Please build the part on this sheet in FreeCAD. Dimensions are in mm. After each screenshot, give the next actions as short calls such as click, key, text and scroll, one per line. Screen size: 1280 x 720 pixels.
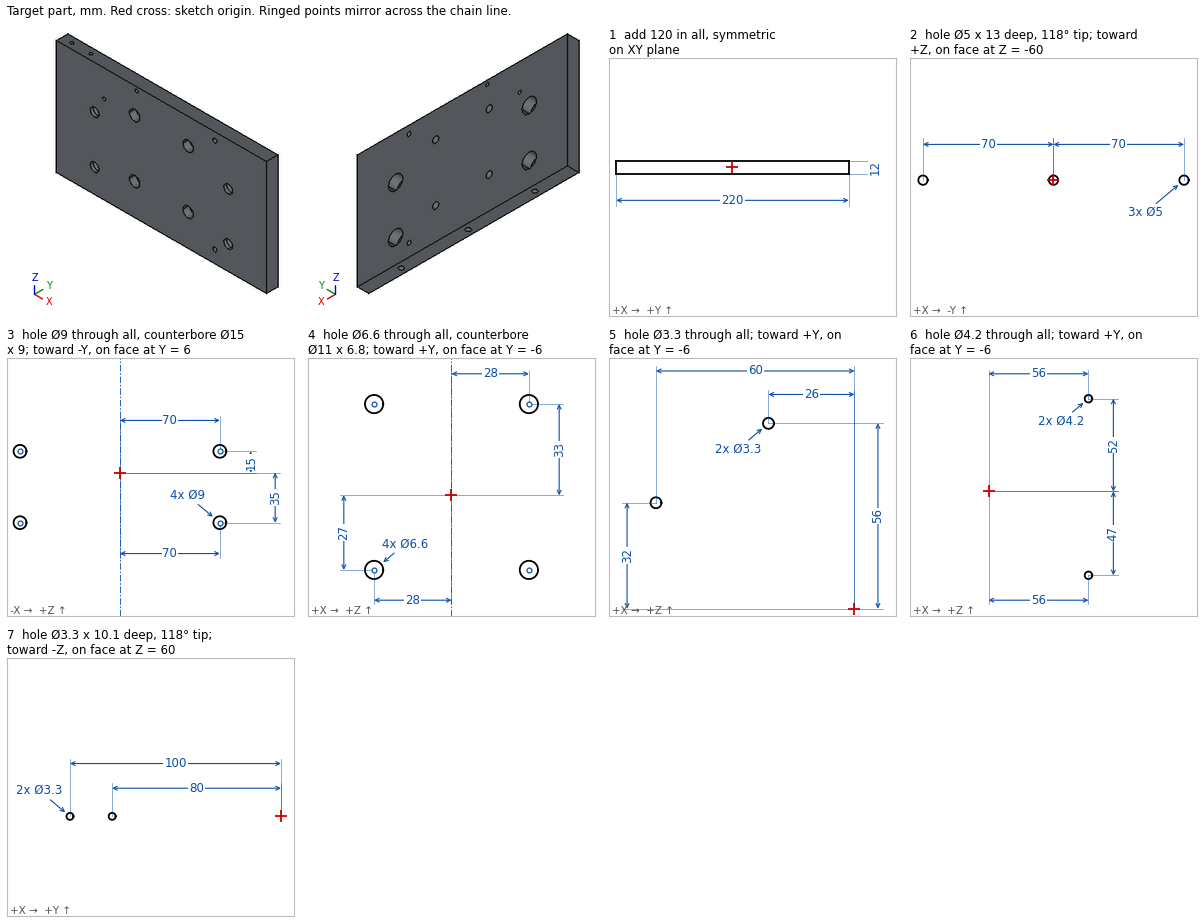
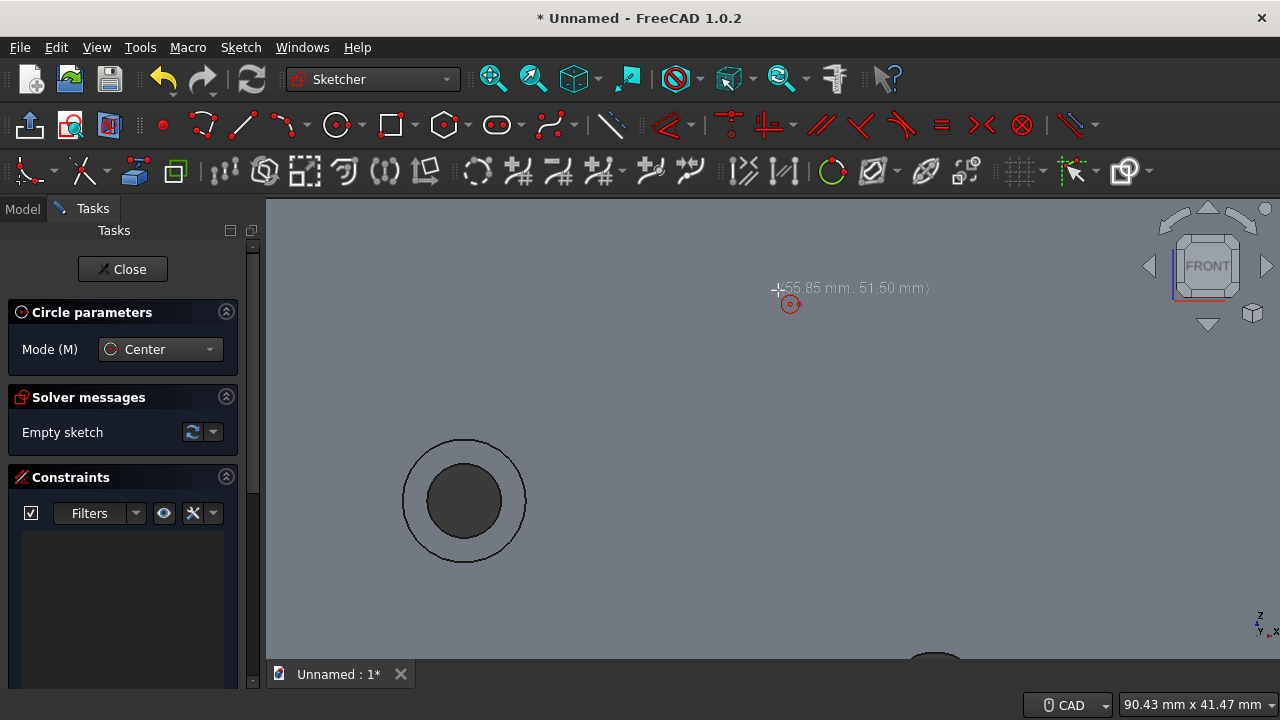
scroll(779, 290, down, 7)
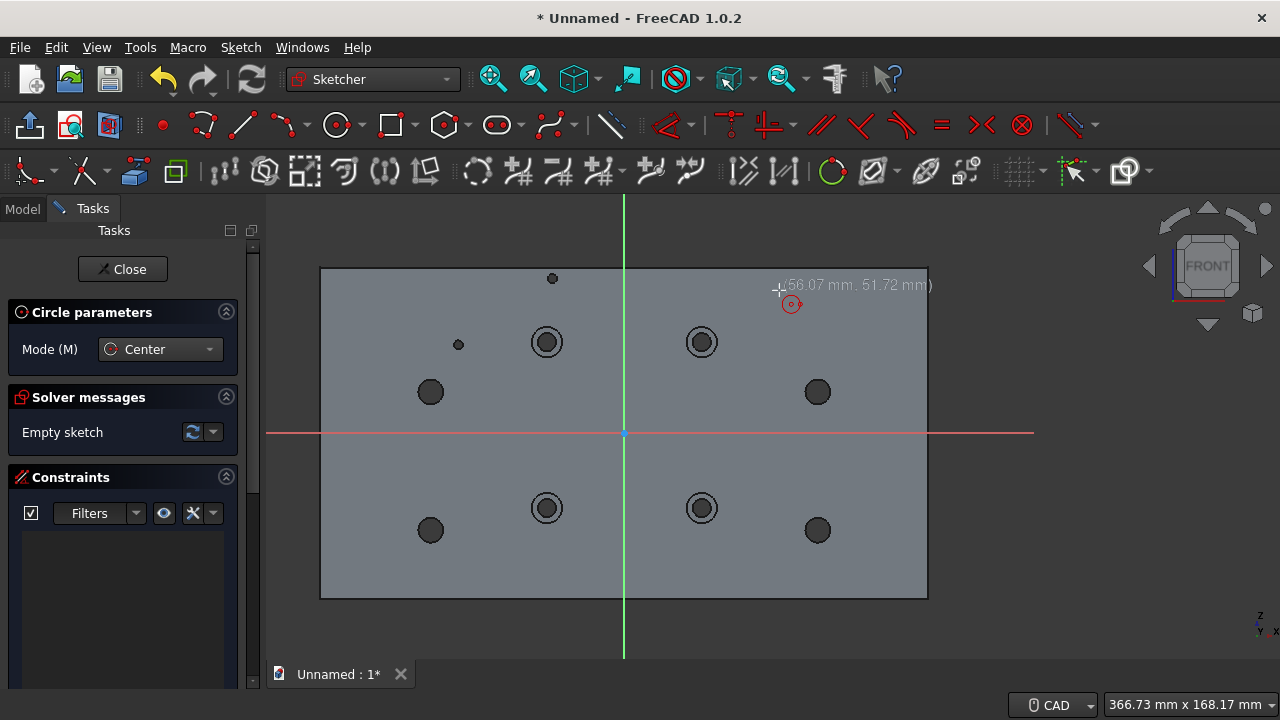
click(779, 290)
move(783, 286)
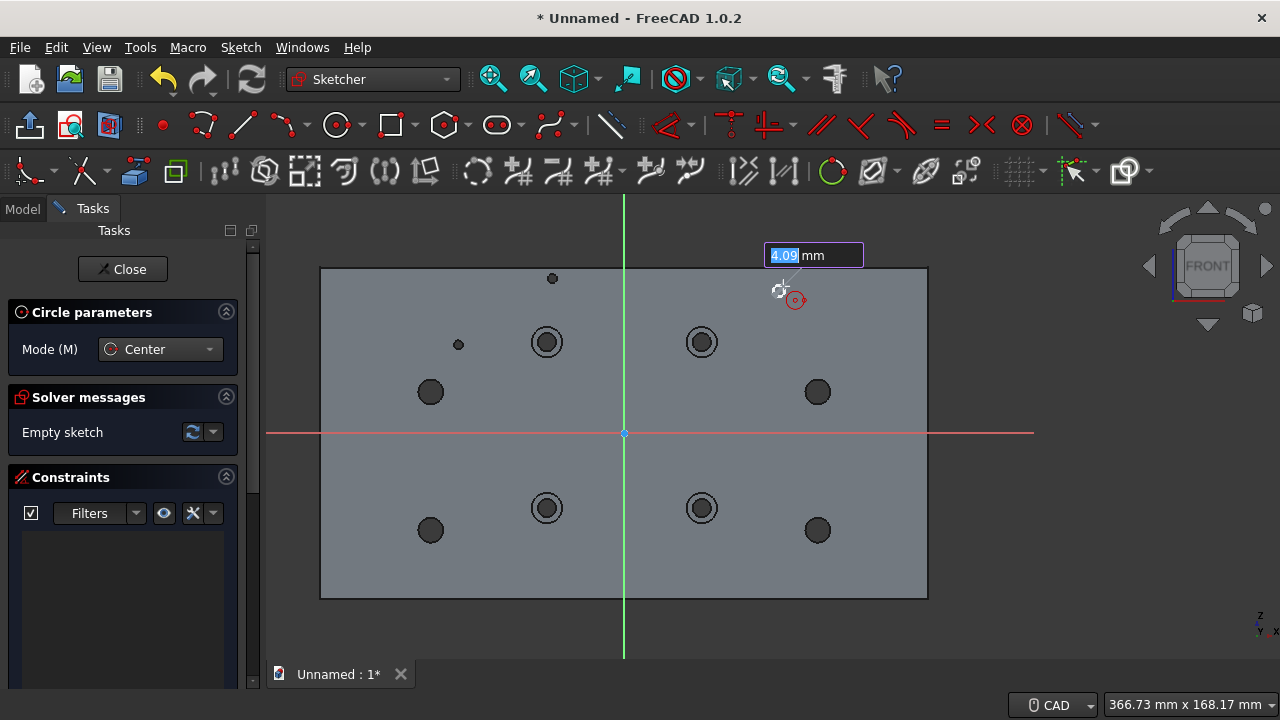
text(4.2)
key(Return)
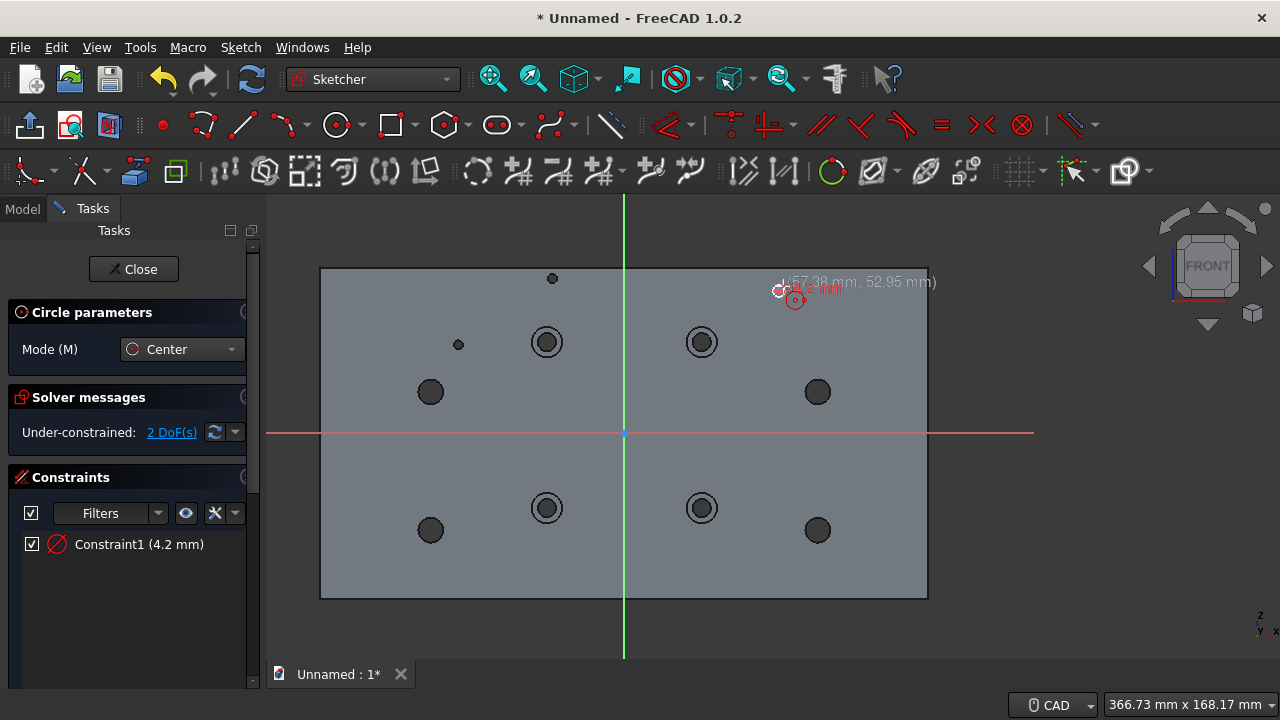
scroll(779, 563, up, 7)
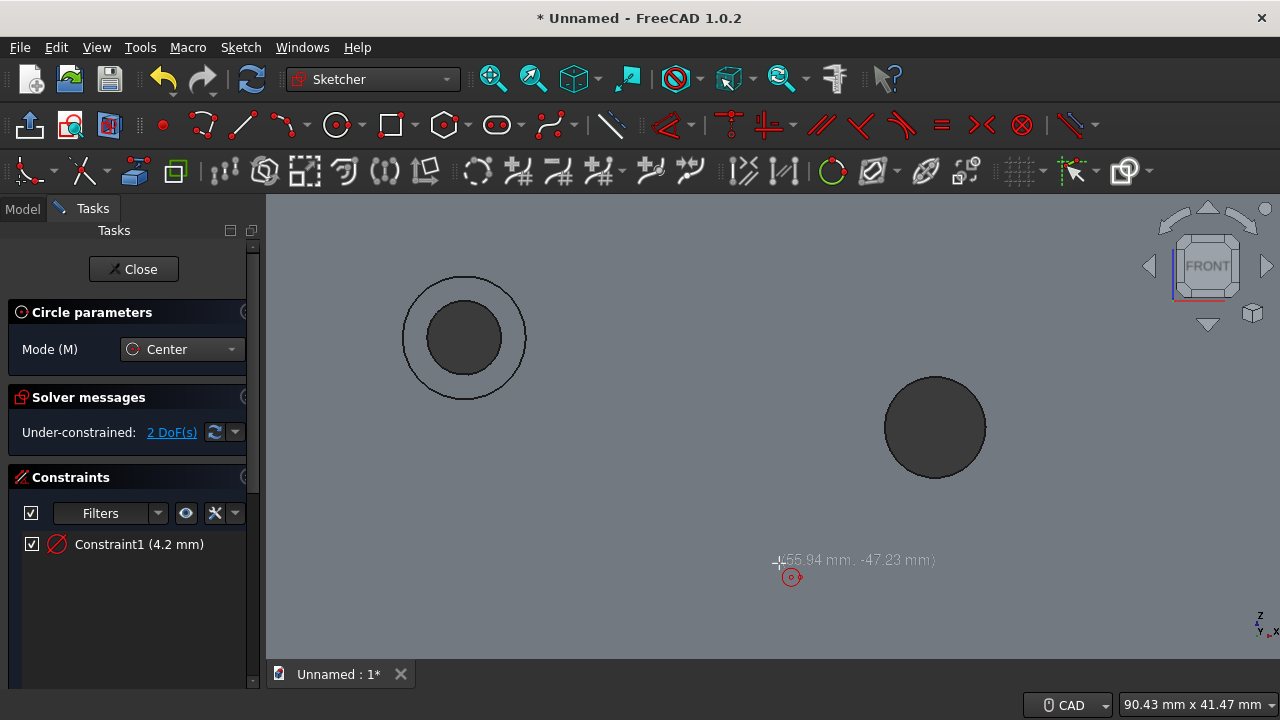
scroll(779, 564, down, 7)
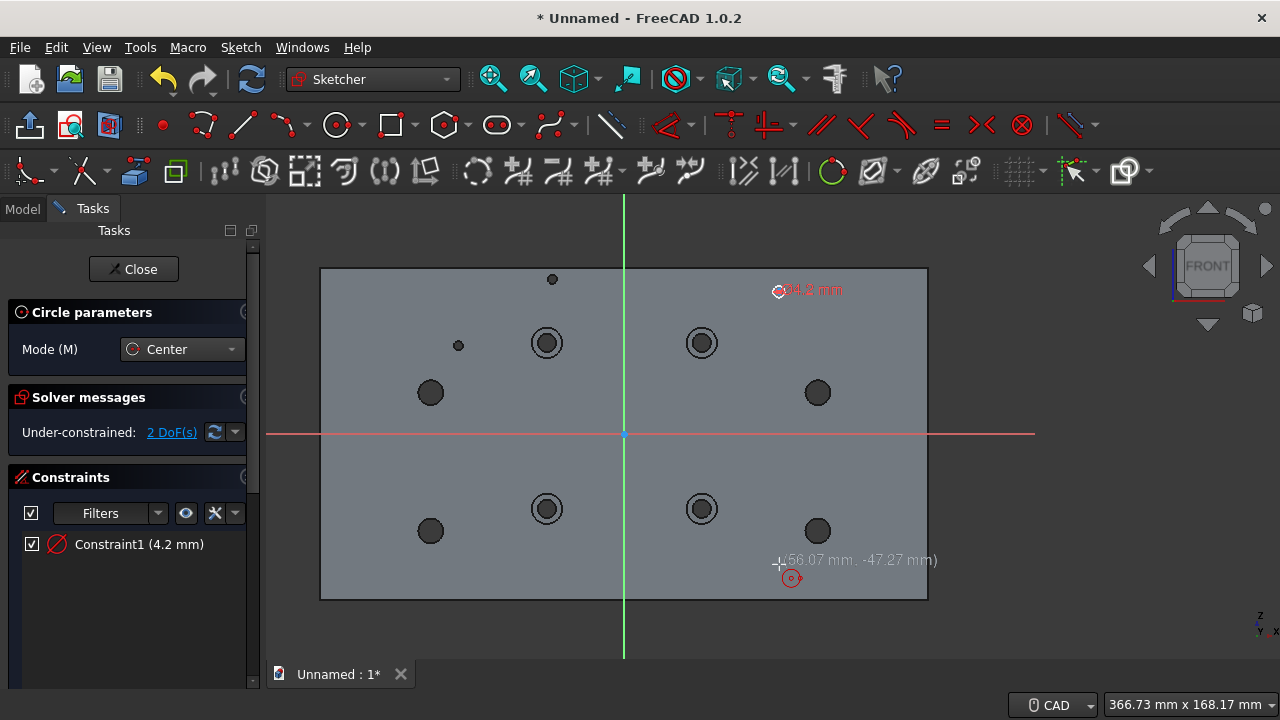
click(779, 564)
move(783, 560)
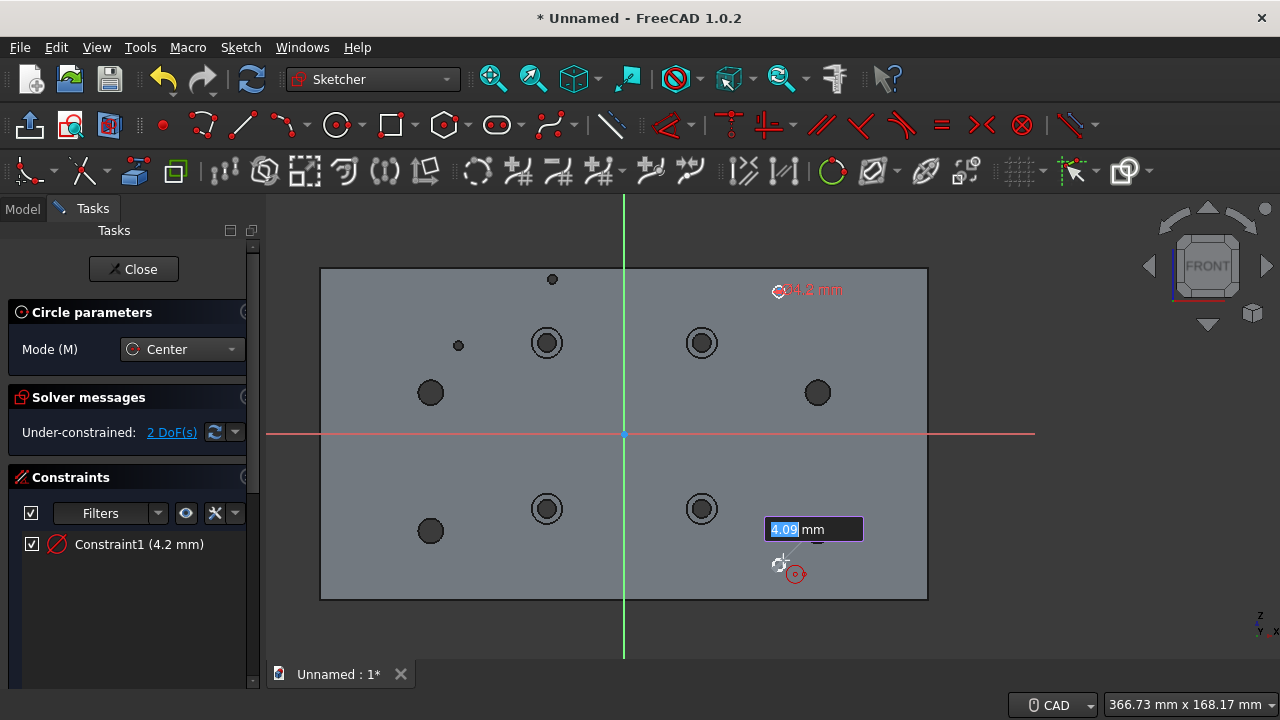
text(4.2)
key(Return)
key(Escape)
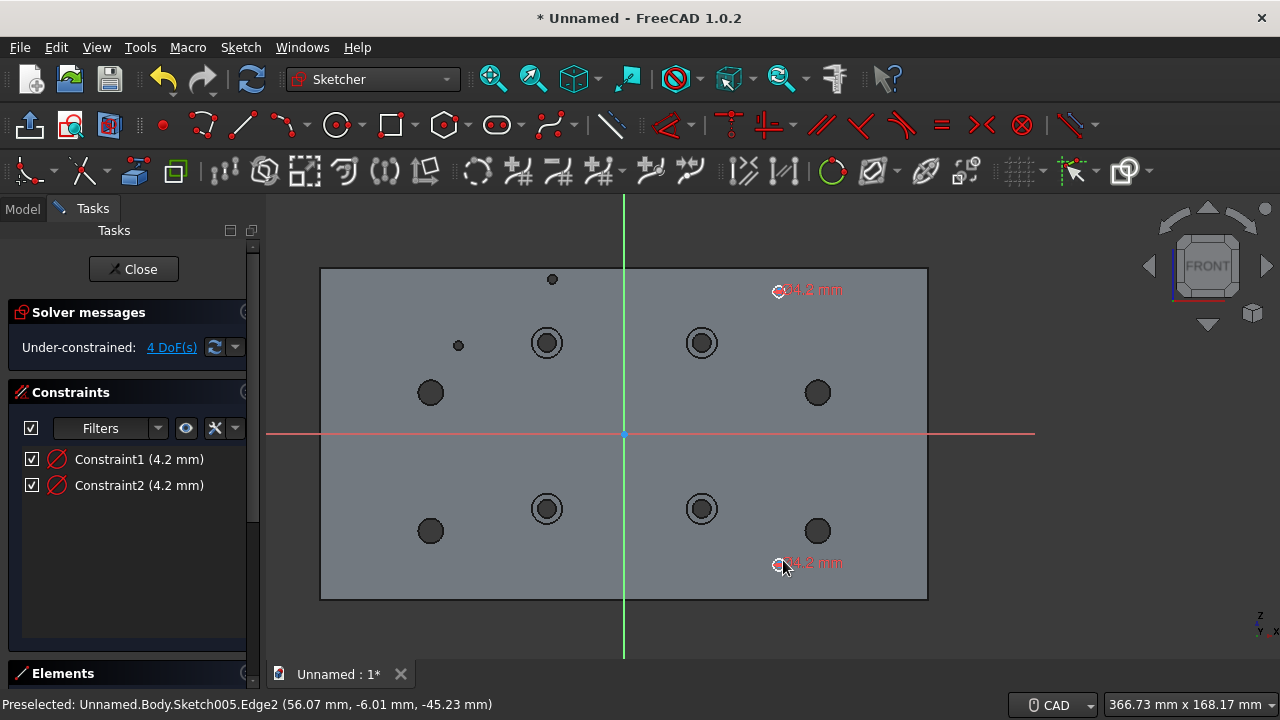
click(666, 126)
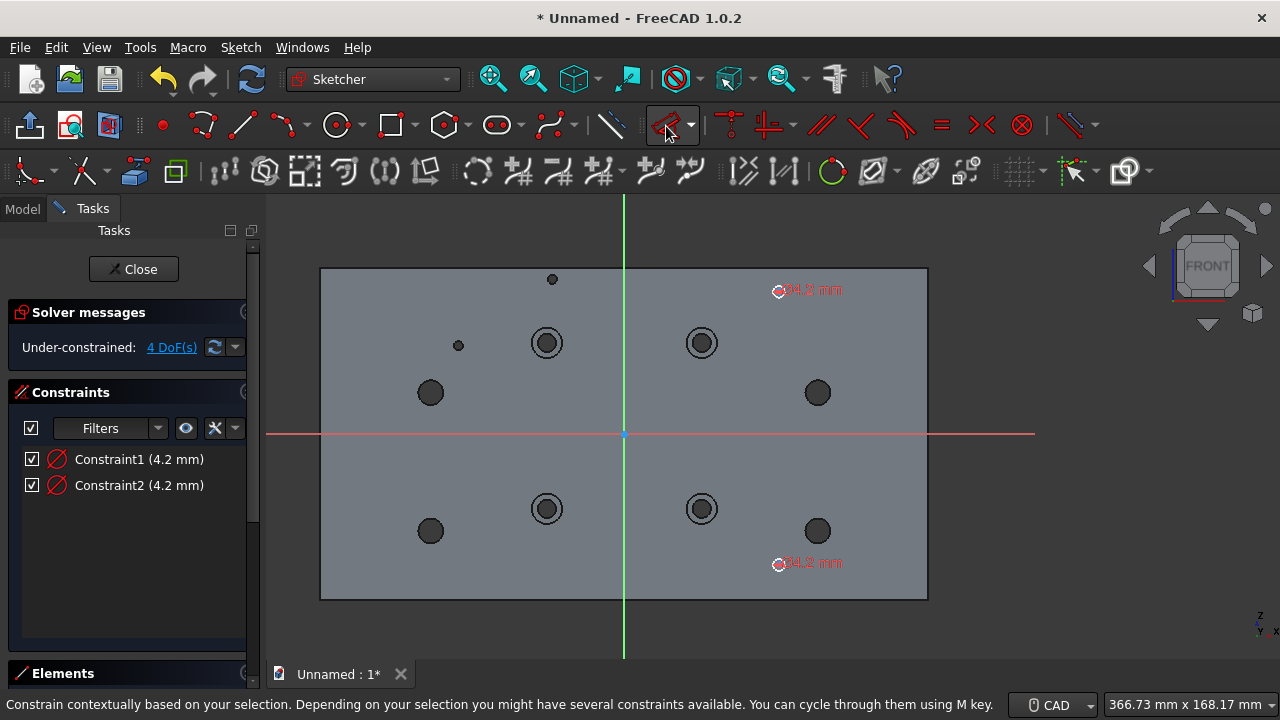
click(779, 292)
click(702, 258)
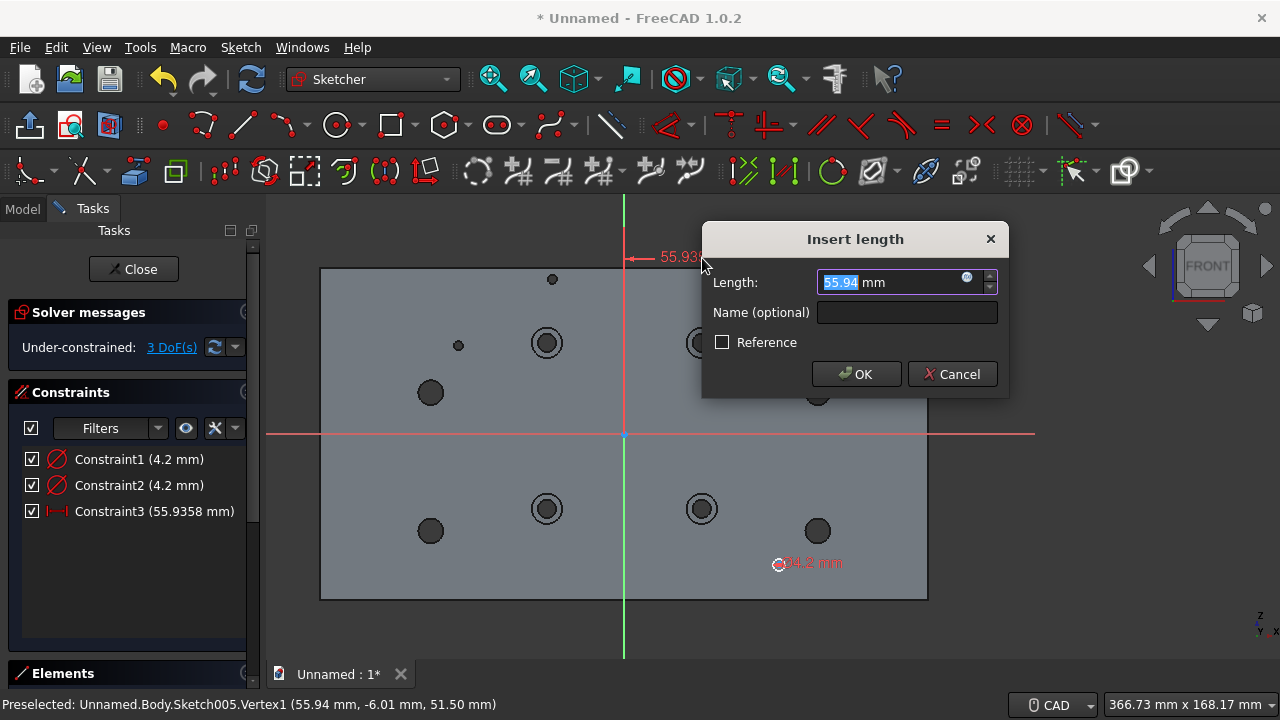
text(56)
key(Return)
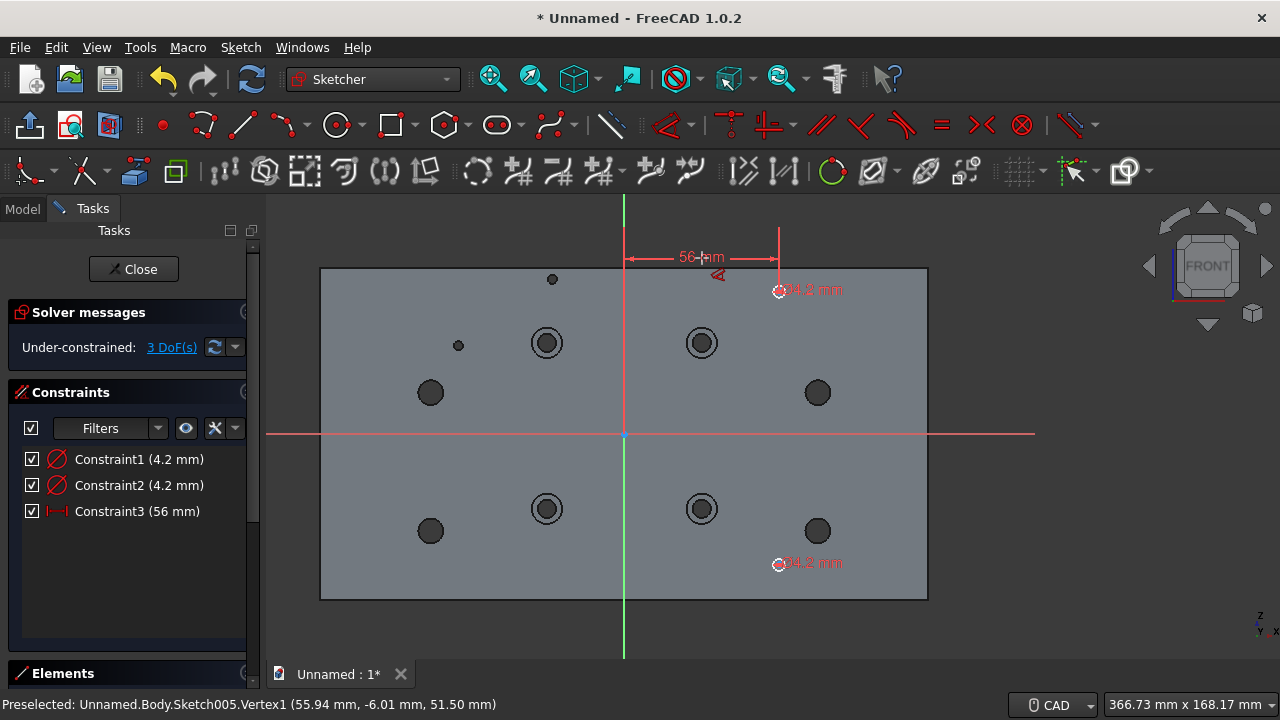
click(779, 292)
click(590, 363)